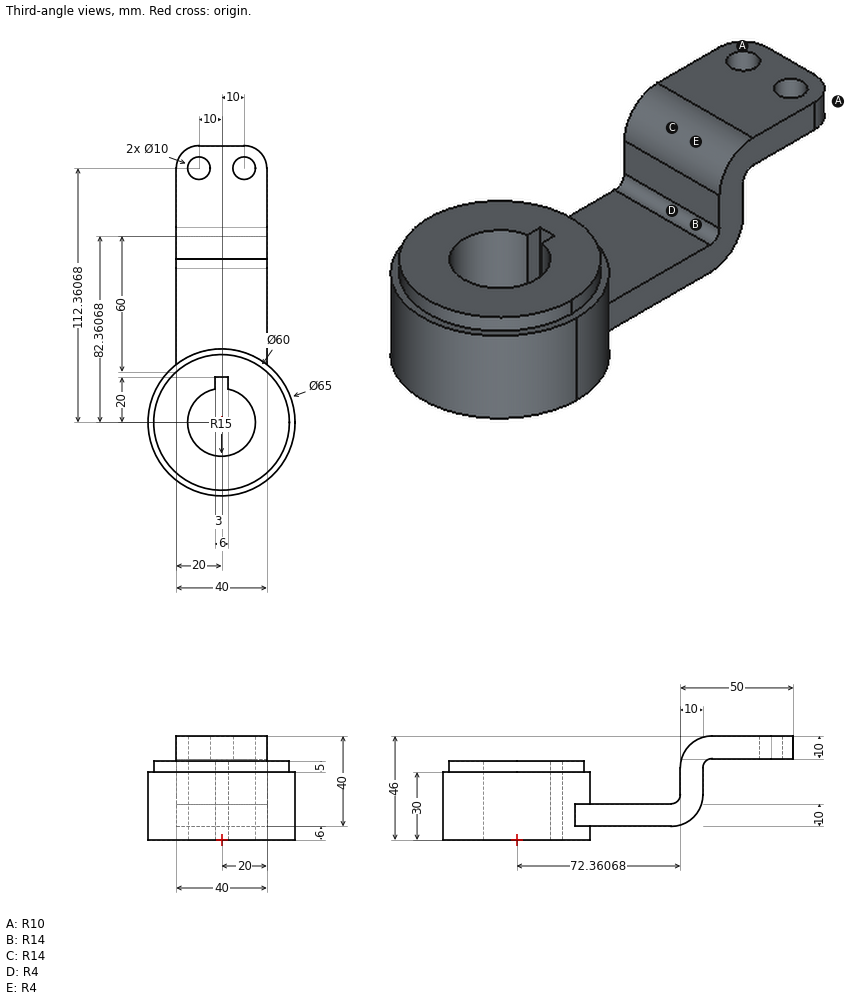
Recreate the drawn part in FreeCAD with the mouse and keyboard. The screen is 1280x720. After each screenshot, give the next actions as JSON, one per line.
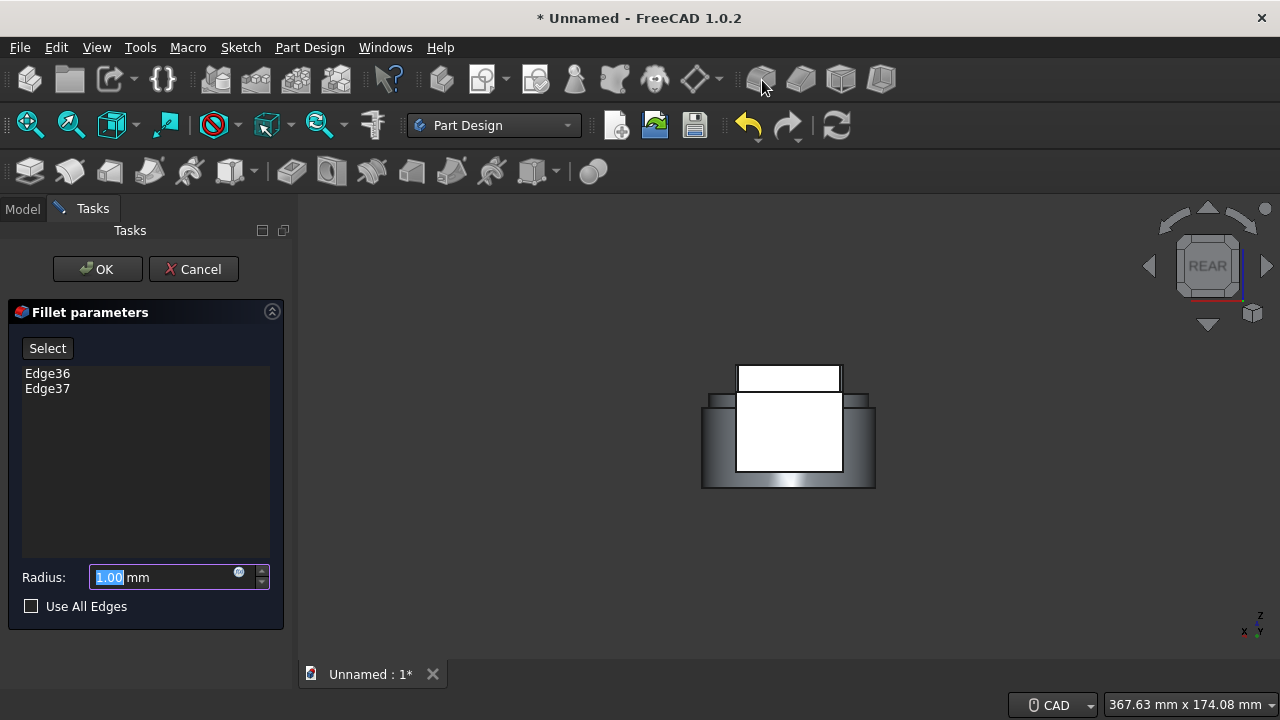
{"action": "type", "text": "10"}
{"action": "key", "text": "Tab"}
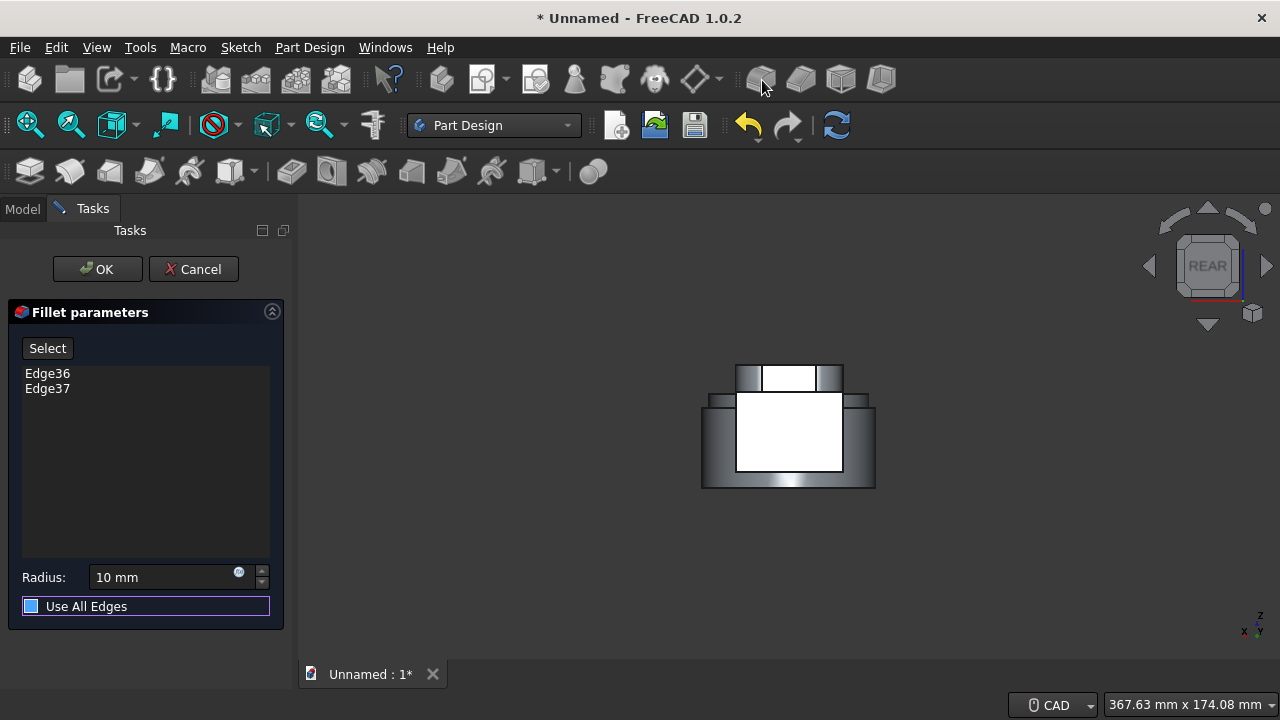
{"action": "left_click", "coordinate": [98, 269]}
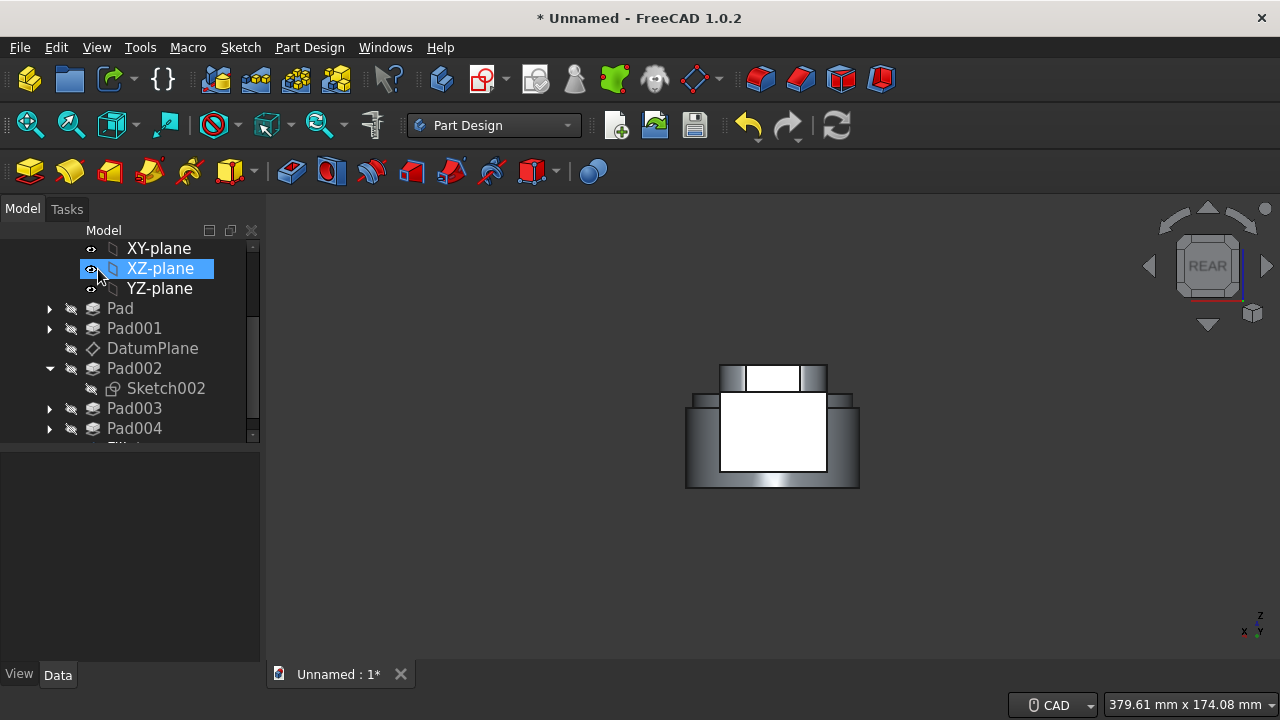
{"action": "key", "text": "v f"}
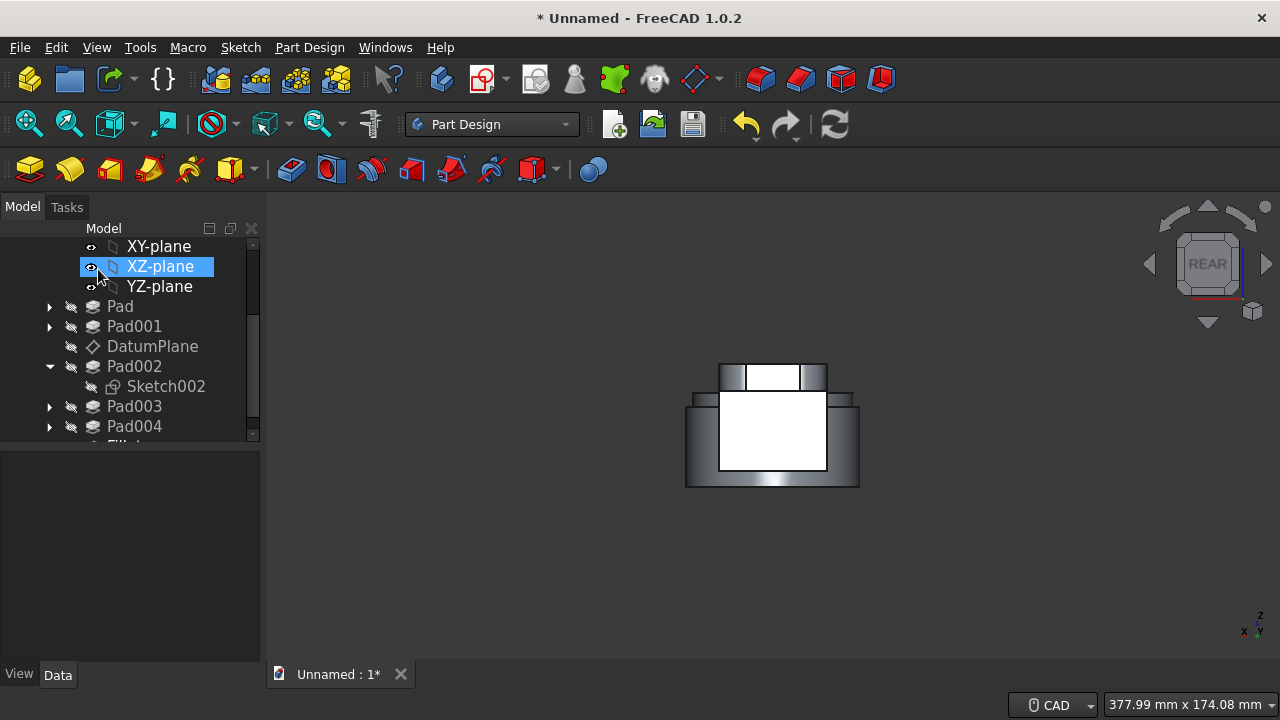
{"action": "left_click", "coordinate": [773, 470]}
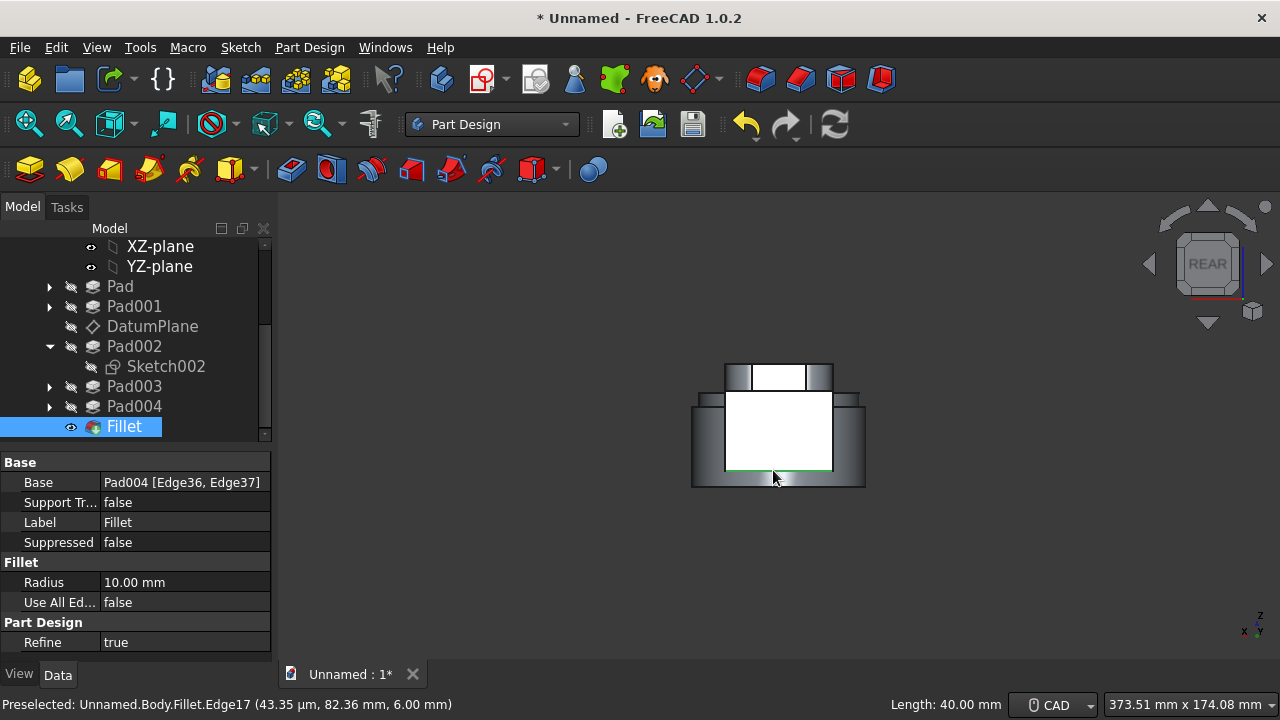
{"action": "left_click", "coordinate": [762, 80]}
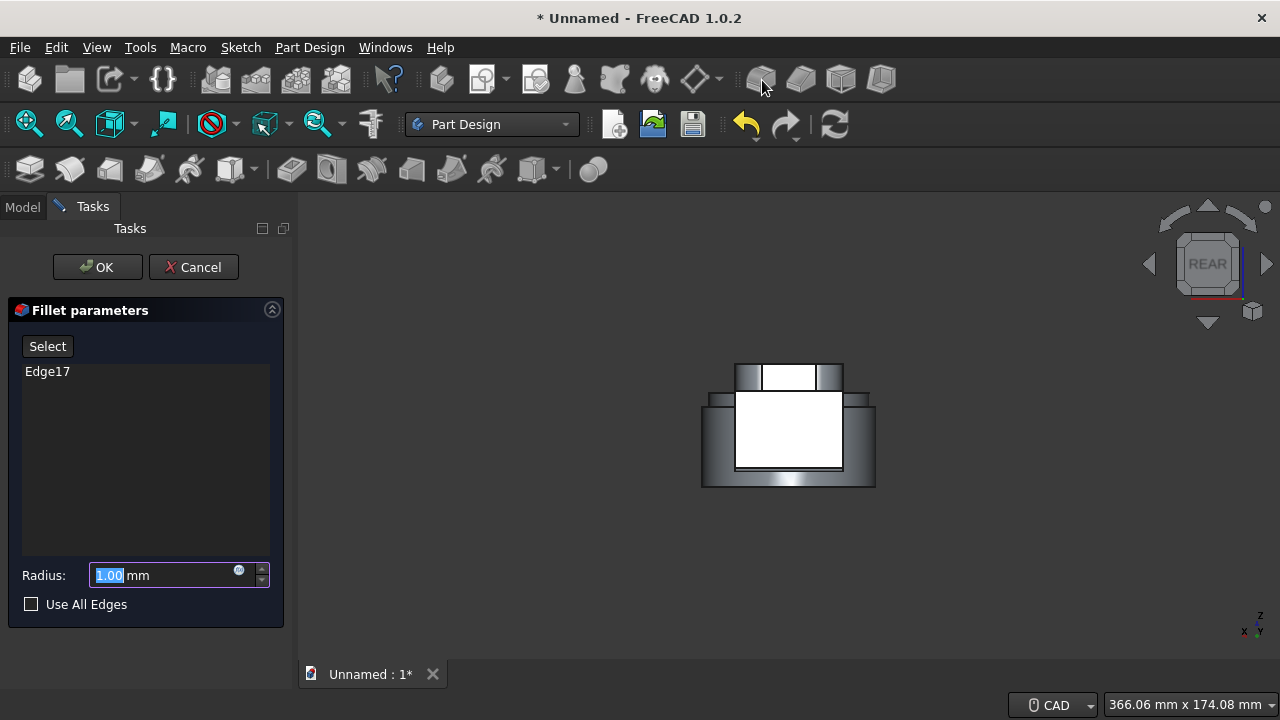
{"action": "type", "text": "14"}
{"action": "key", "text": "Tab"}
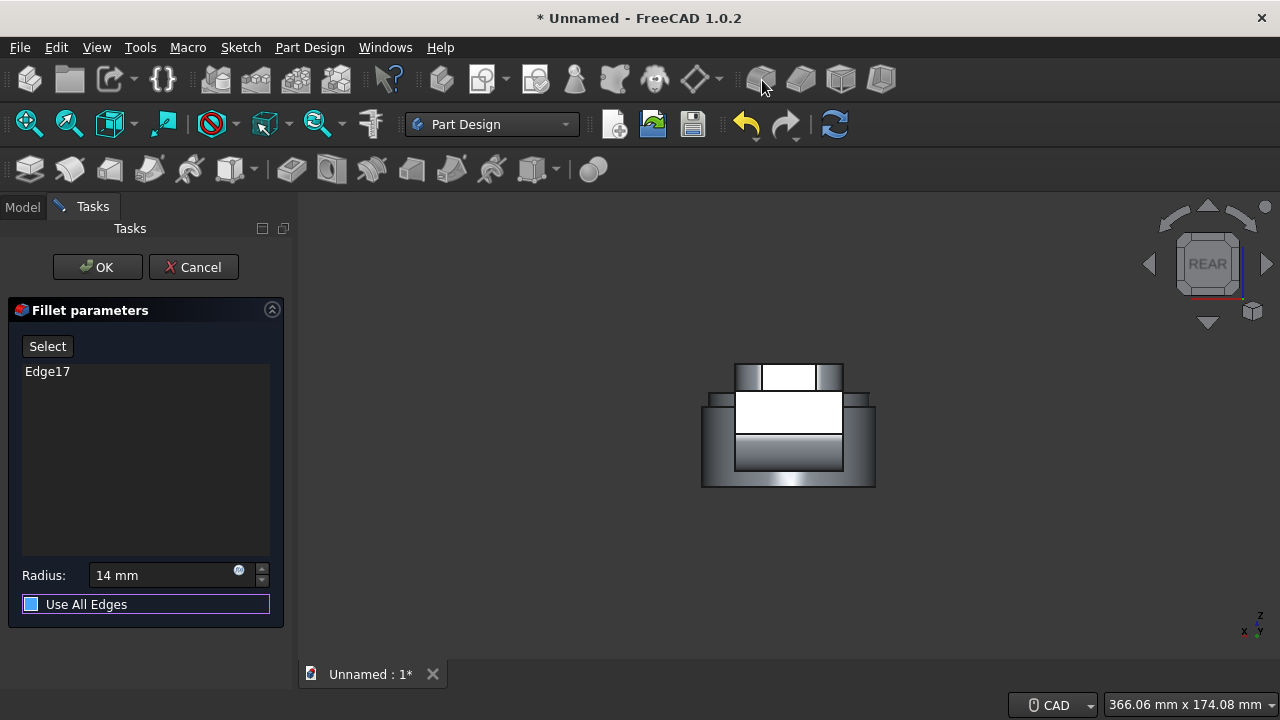
{"action": "left_click", "coordinate": [98, 267]}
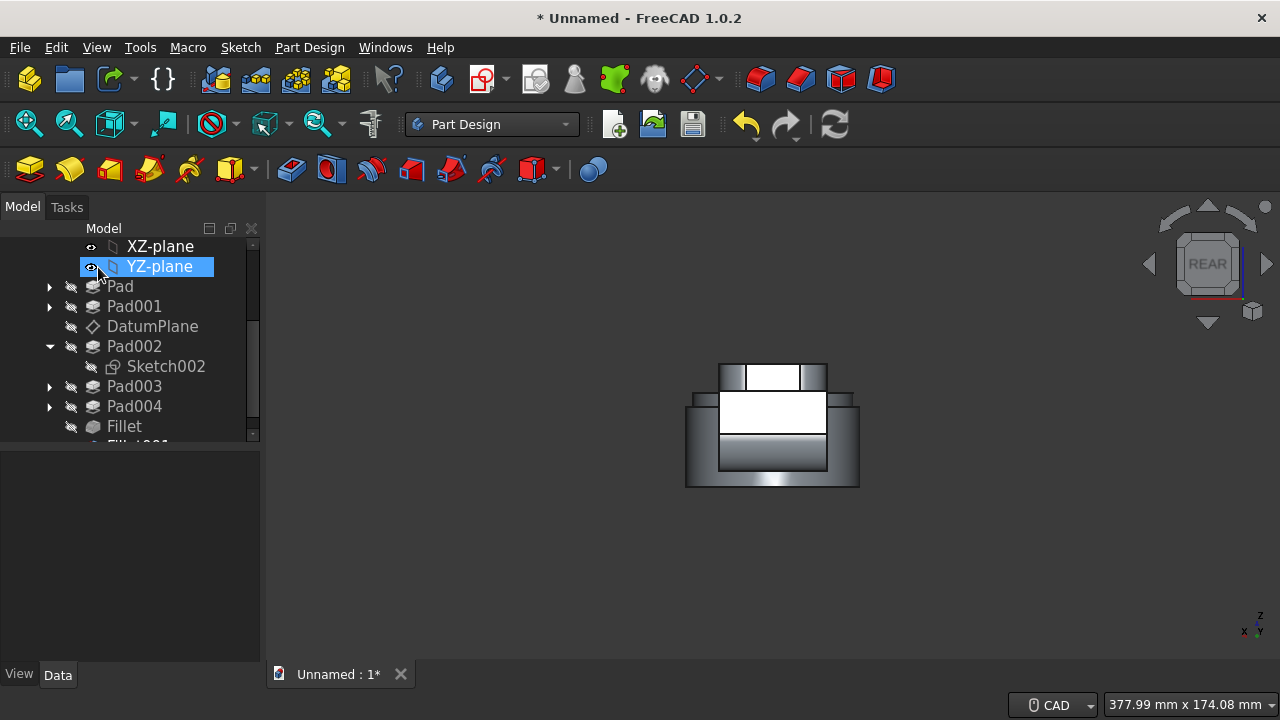
{"action": "left_click", "coordinate": [30, 124]}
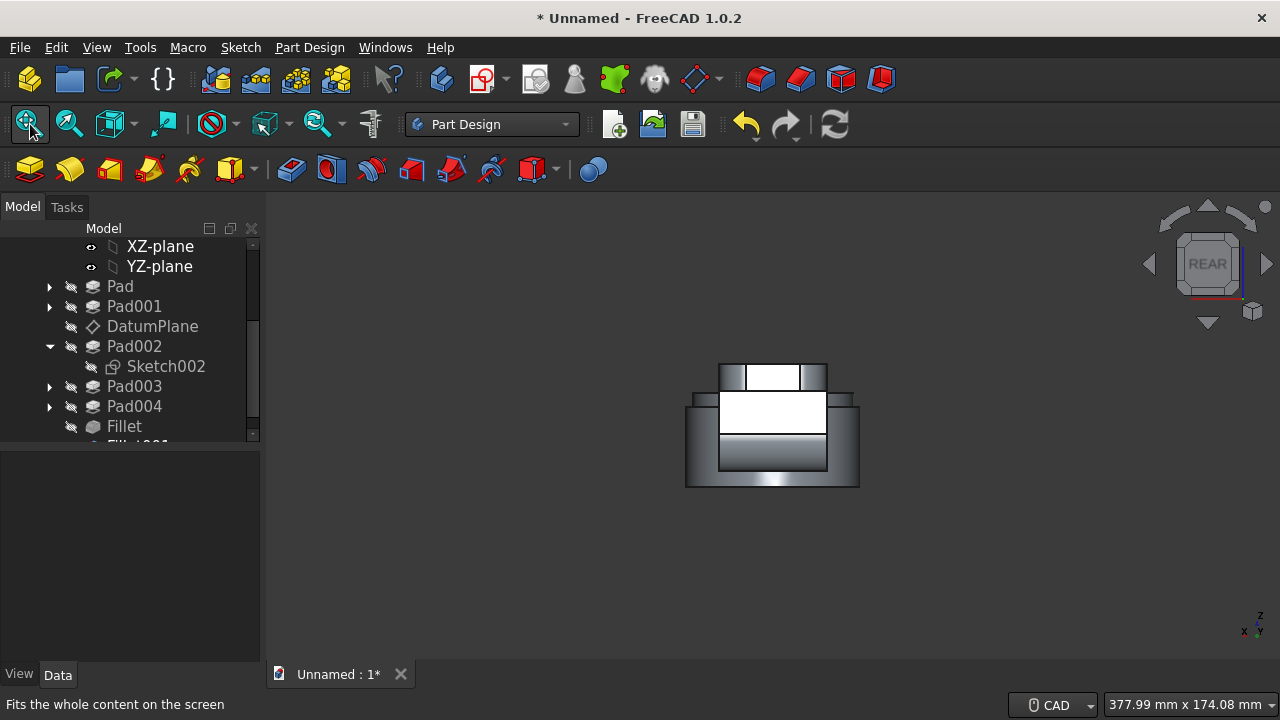
{"action": "key", "text": "0"}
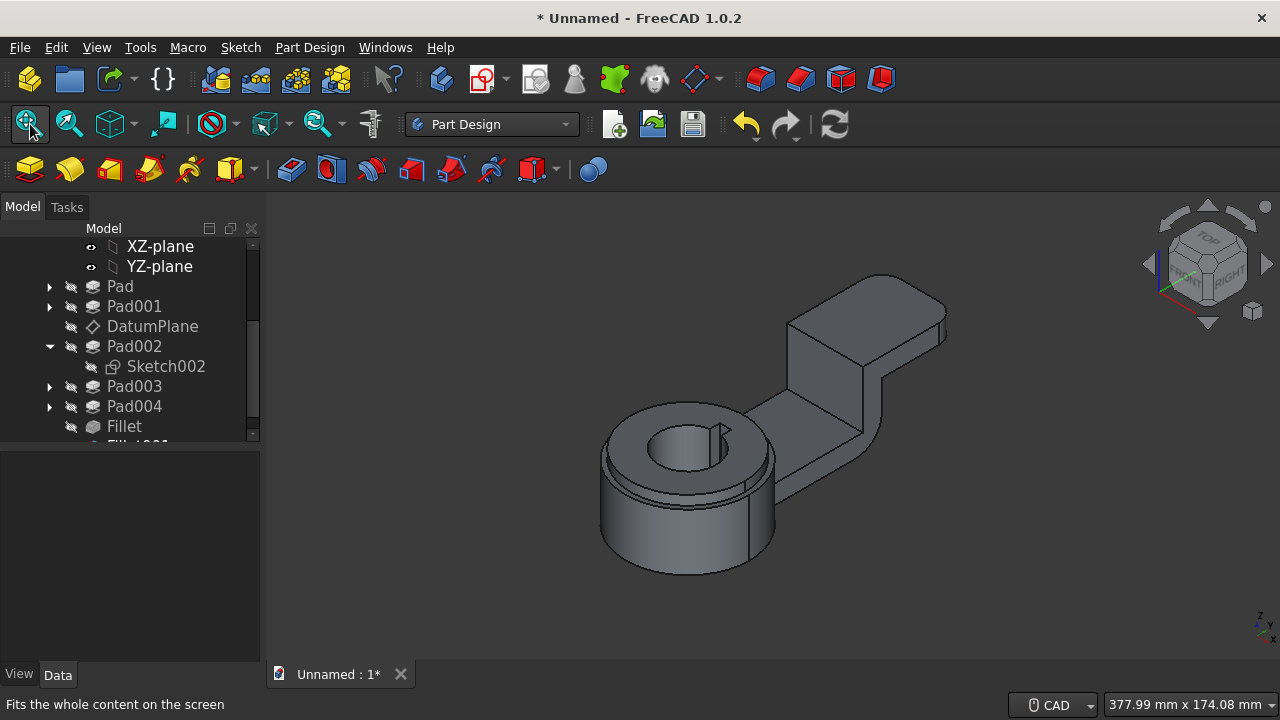
{"action": "left_click", "coordinate": [825, 344]}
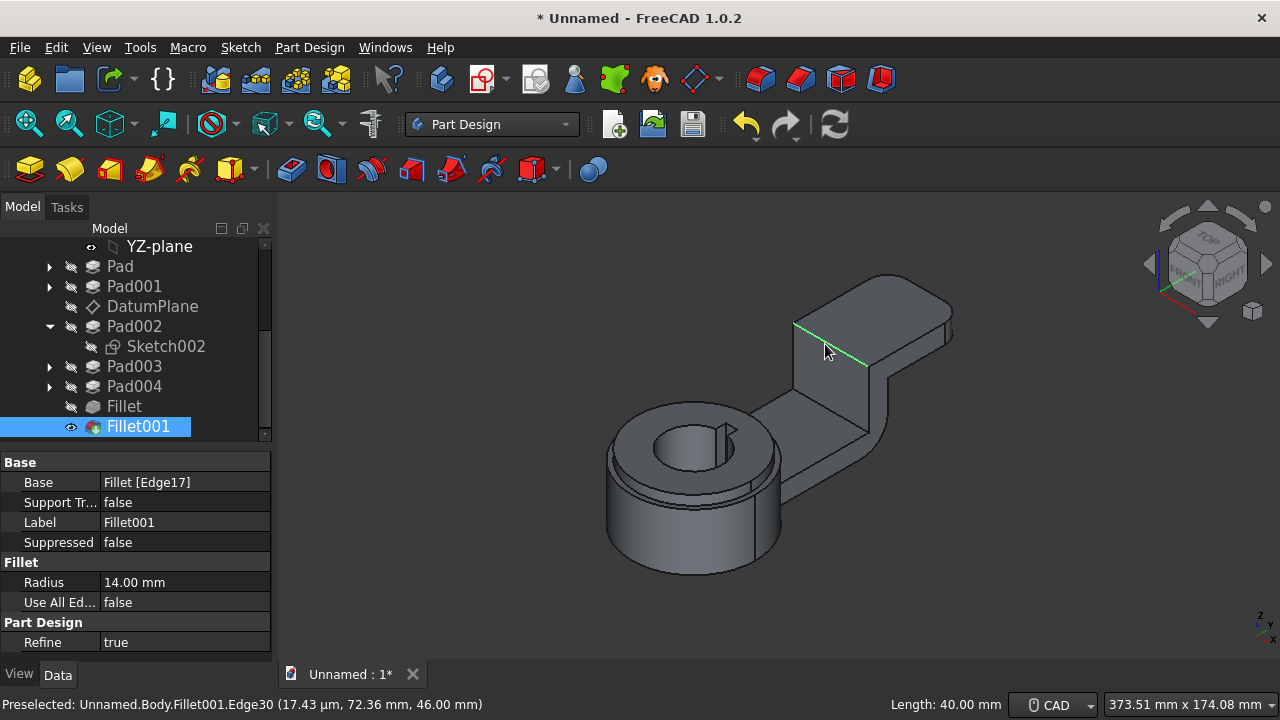
{"action": "left_click", "coordinate": [762, 80]}